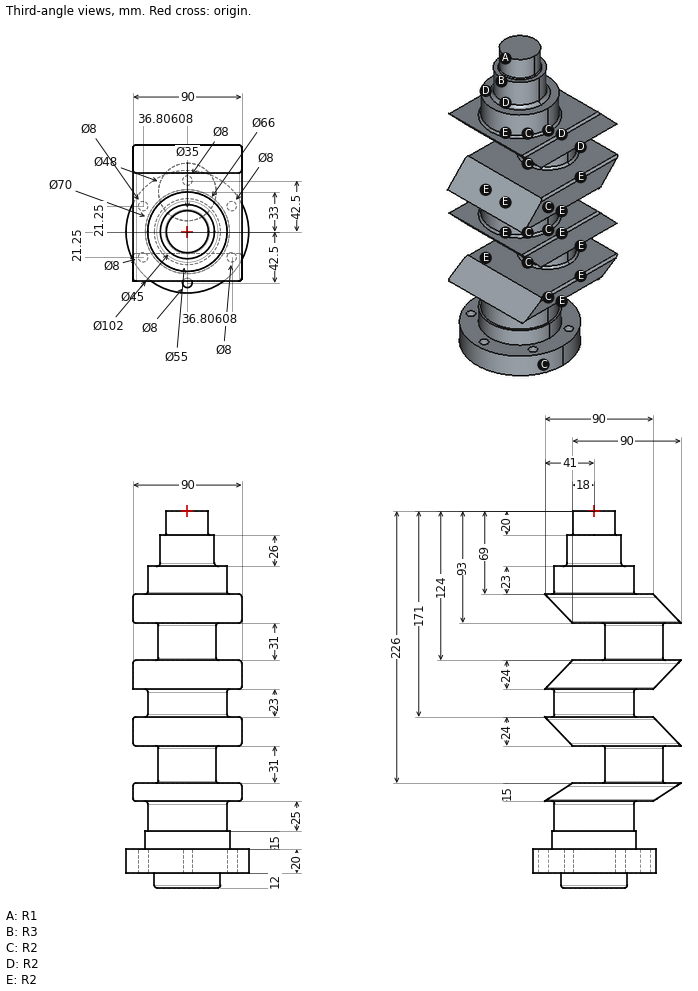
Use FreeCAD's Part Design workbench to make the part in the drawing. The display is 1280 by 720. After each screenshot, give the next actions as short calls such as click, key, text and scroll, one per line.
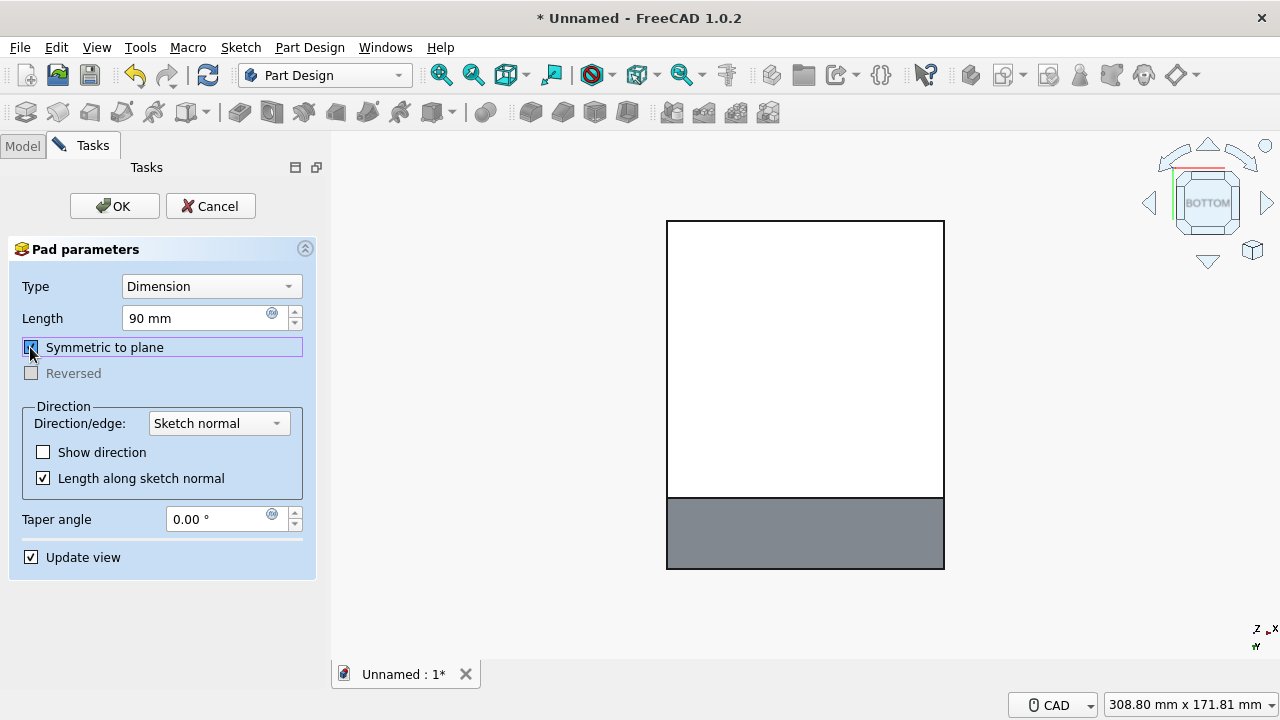
click(115, 206)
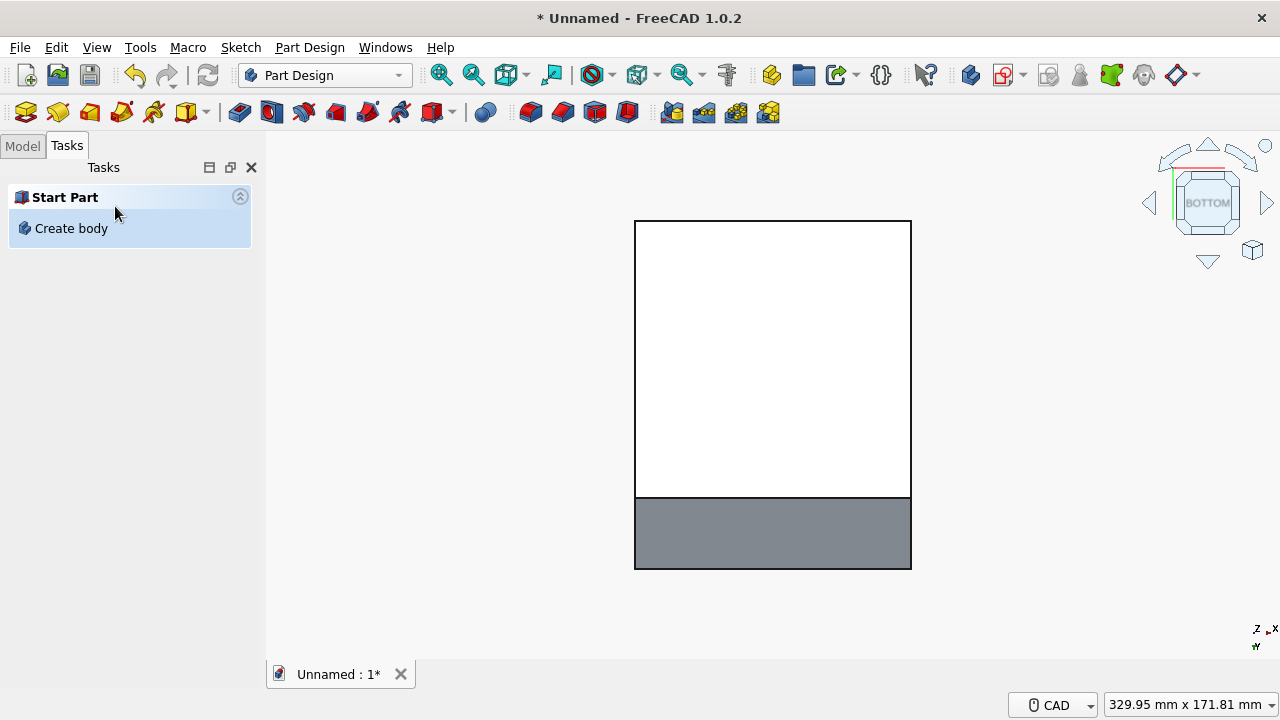
click(773, 359)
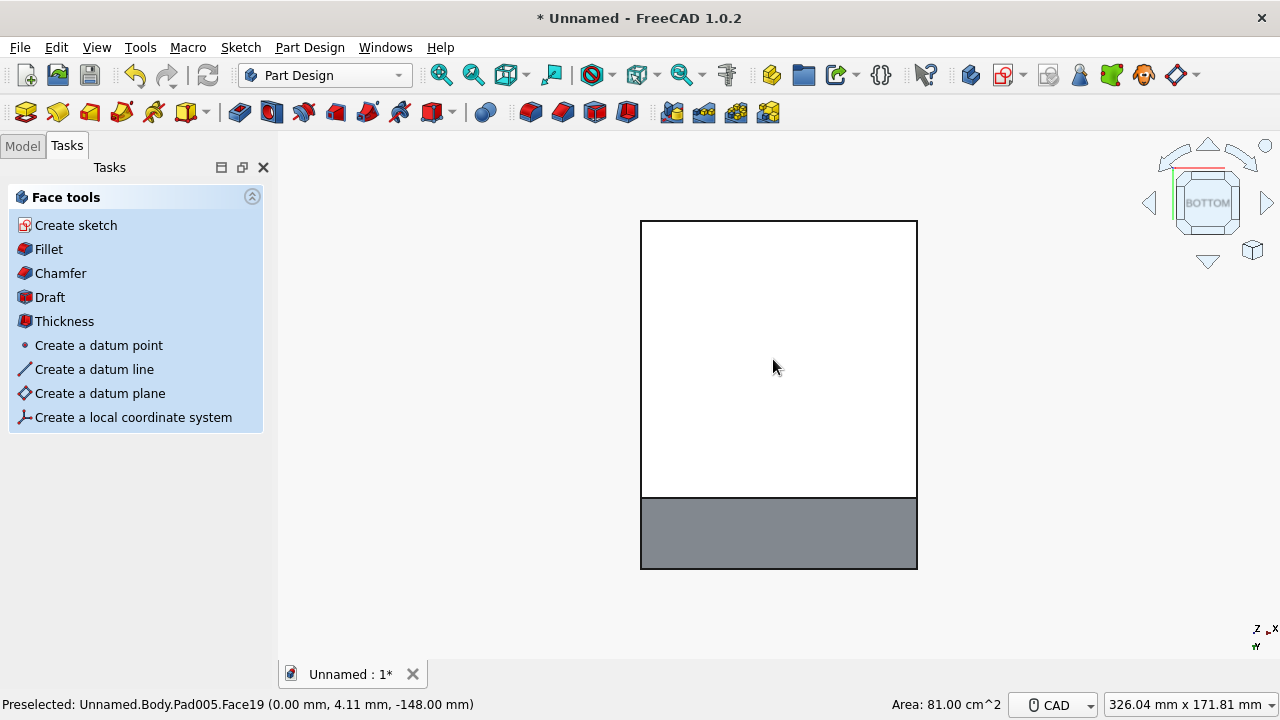
click(1004, 76)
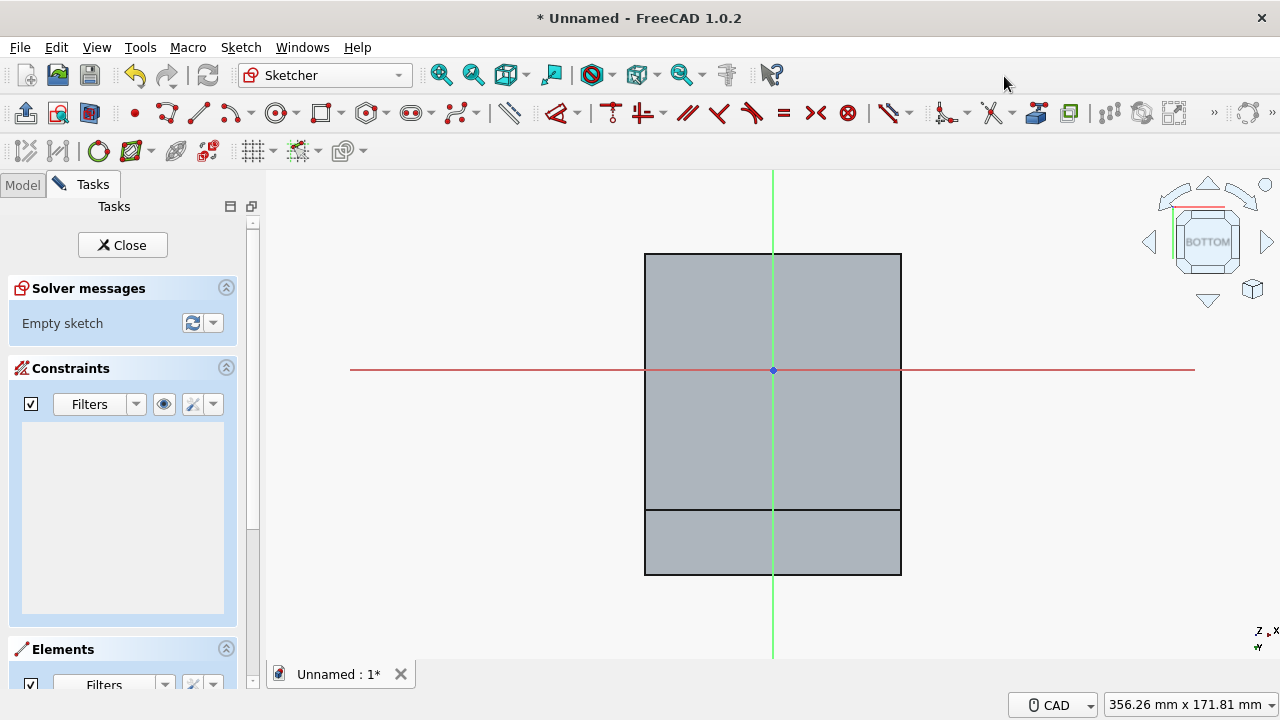
scroll(912, 281, up, 2)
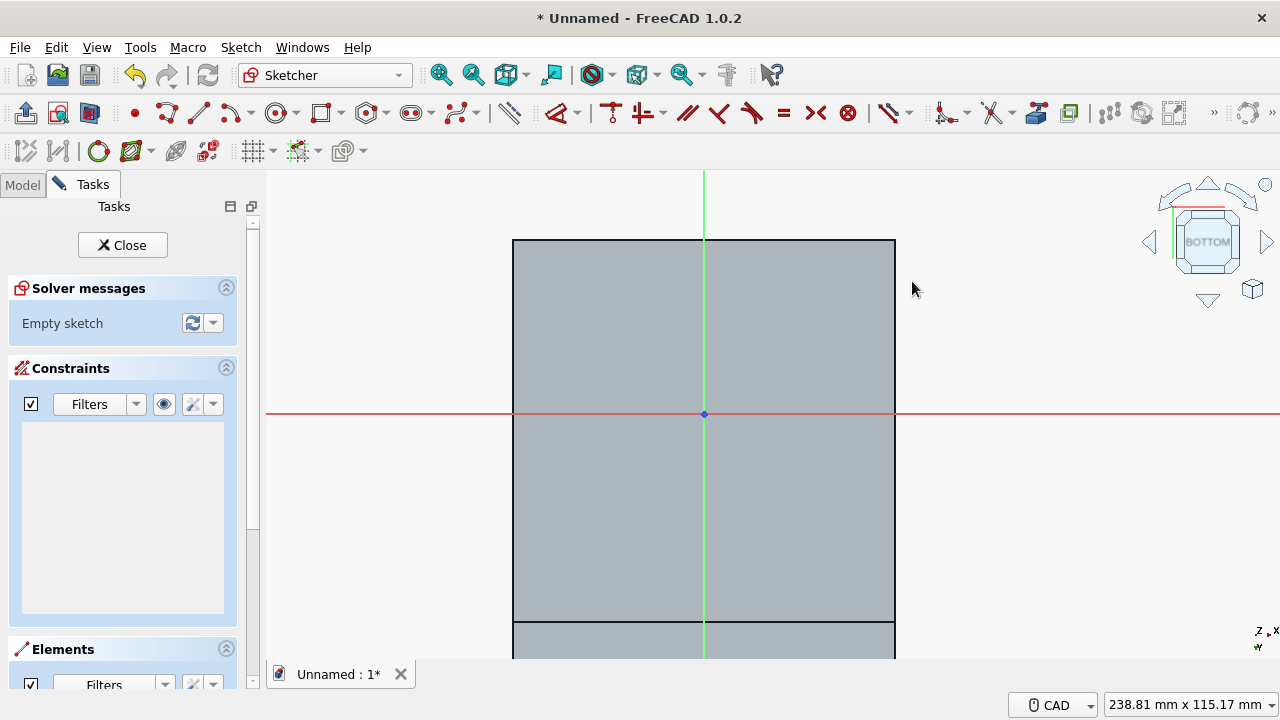
click(276, 114)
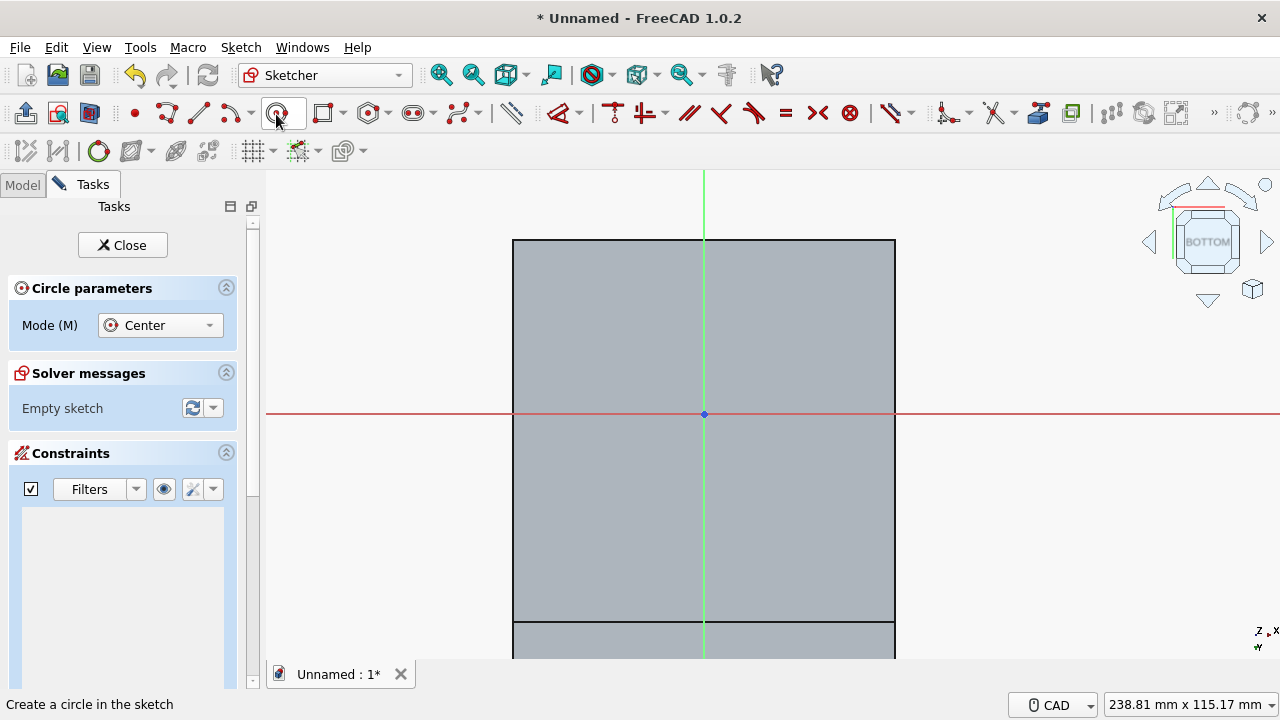
click(704, 414)
move(803, 315)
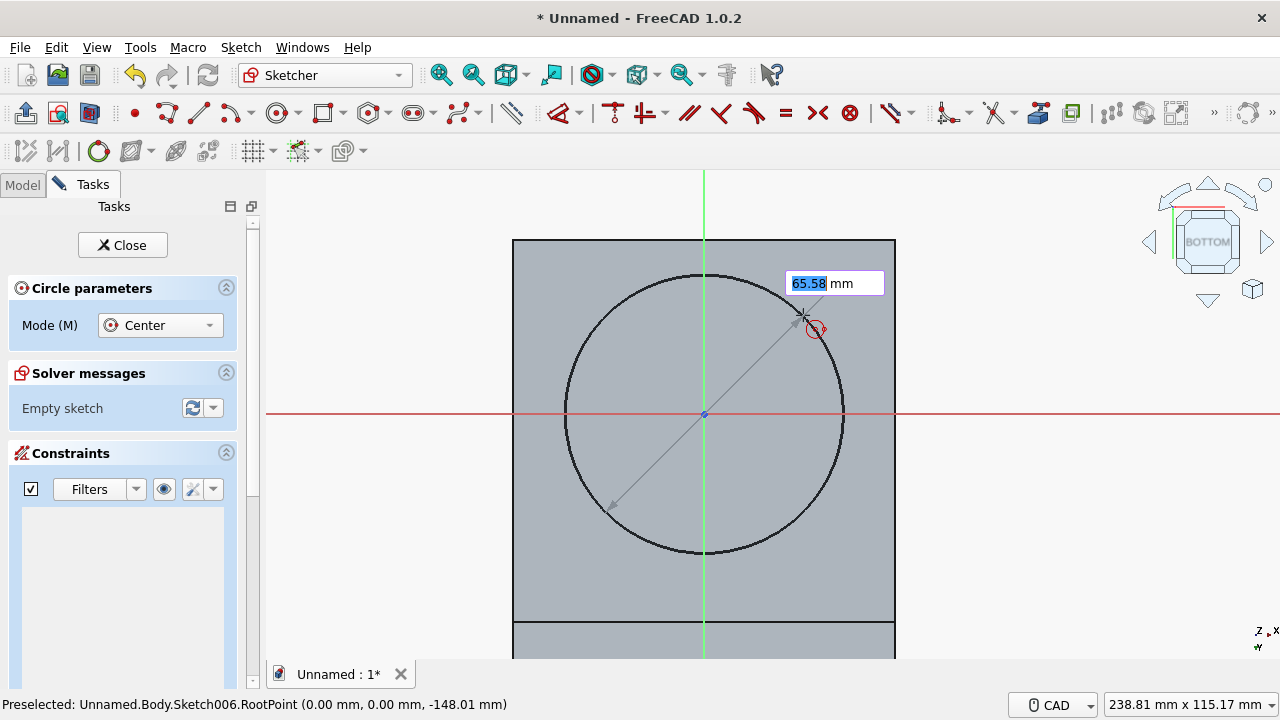
text(66)
key(Return)
key(Escape)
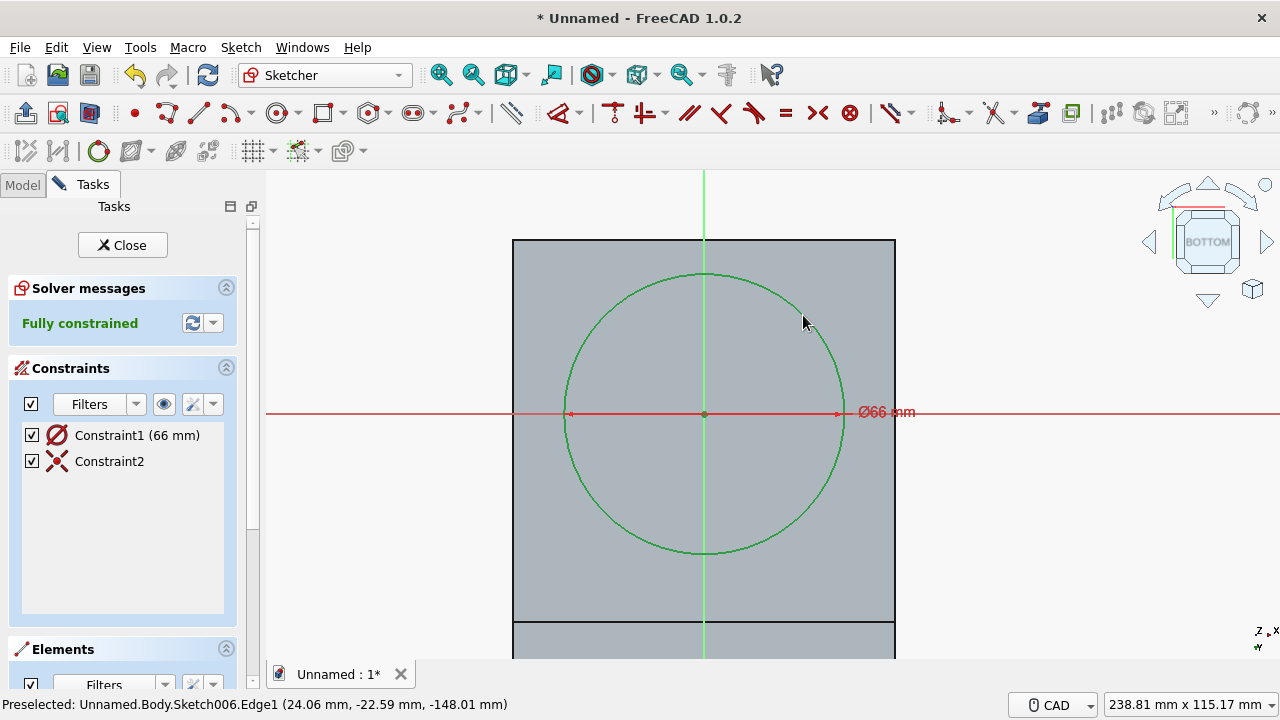
click(123, 245)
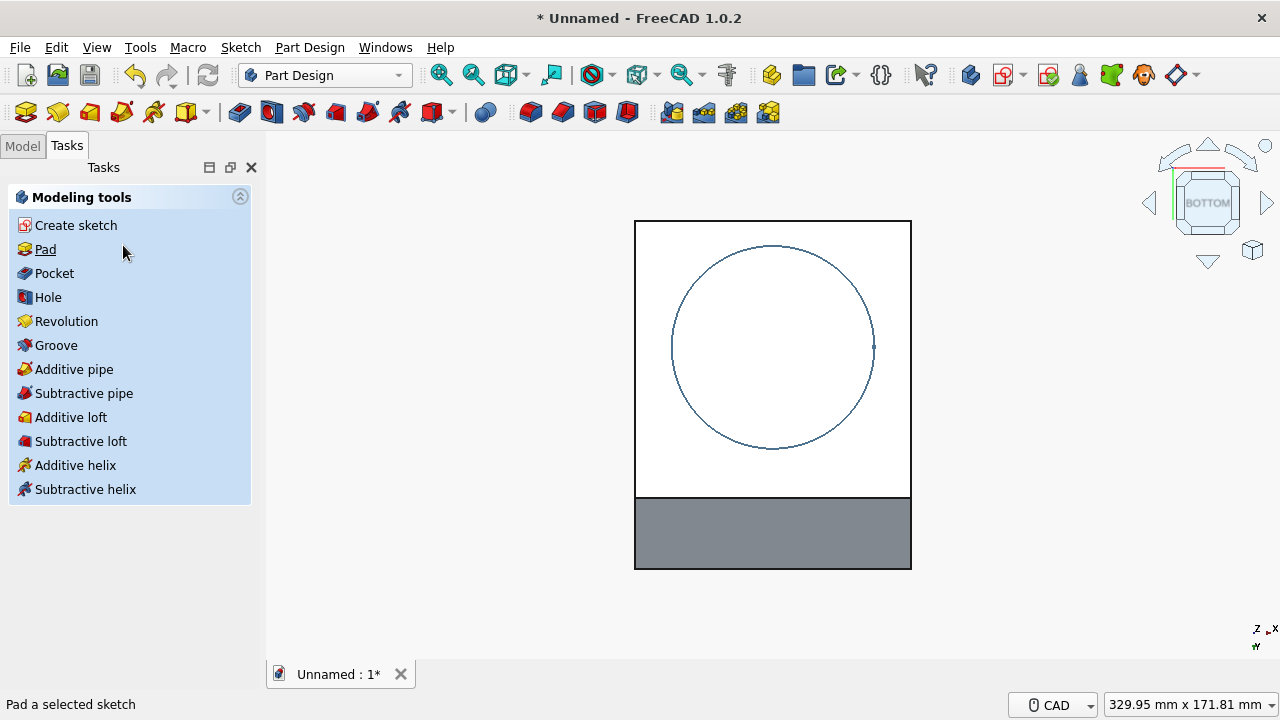
click(26, 112)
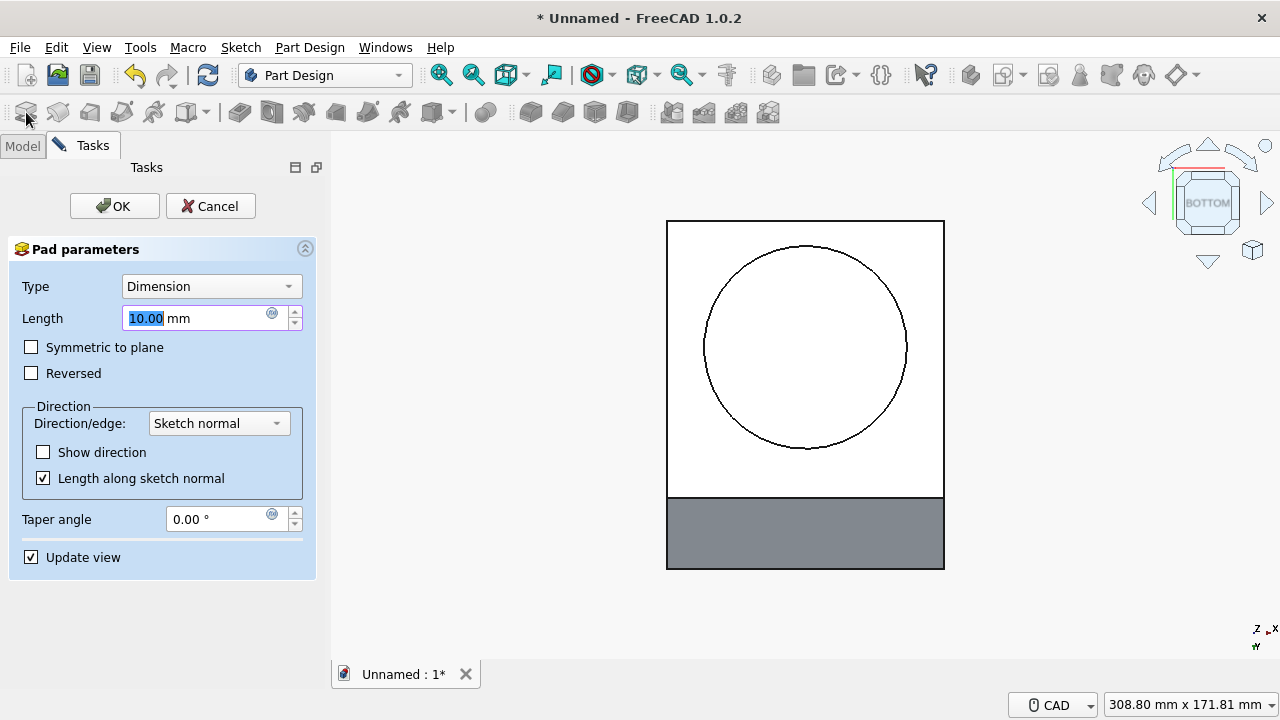
text(23)
key(Tab)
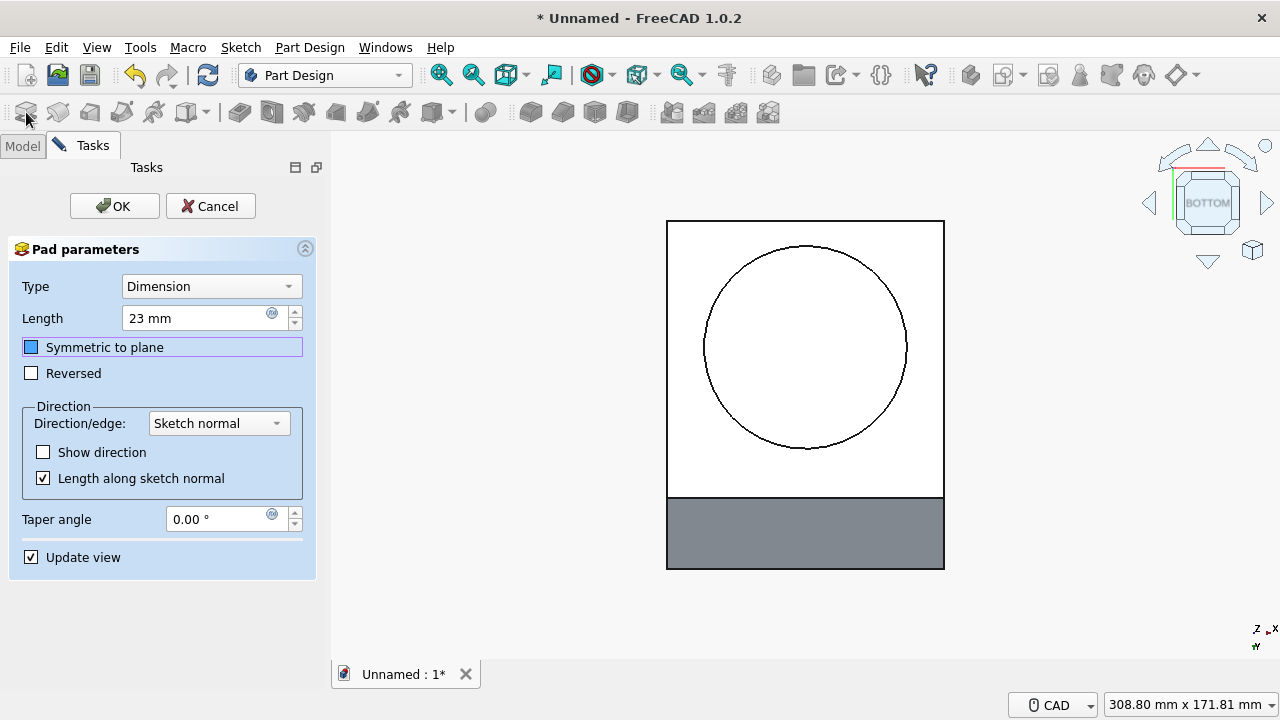
click(115, 206)